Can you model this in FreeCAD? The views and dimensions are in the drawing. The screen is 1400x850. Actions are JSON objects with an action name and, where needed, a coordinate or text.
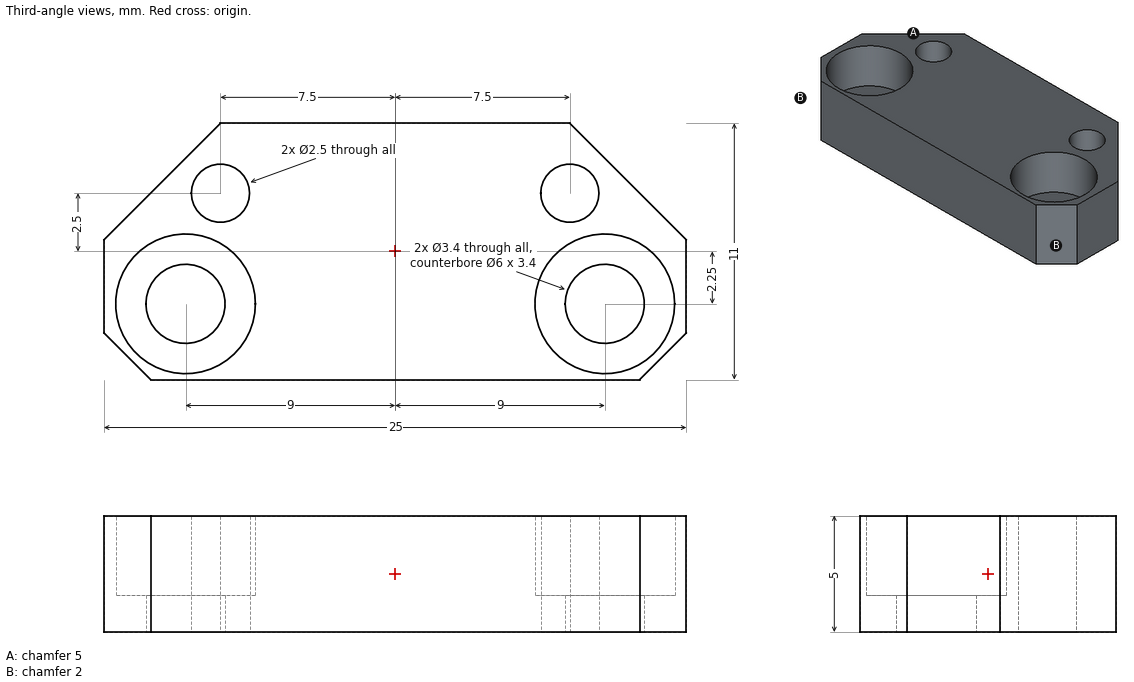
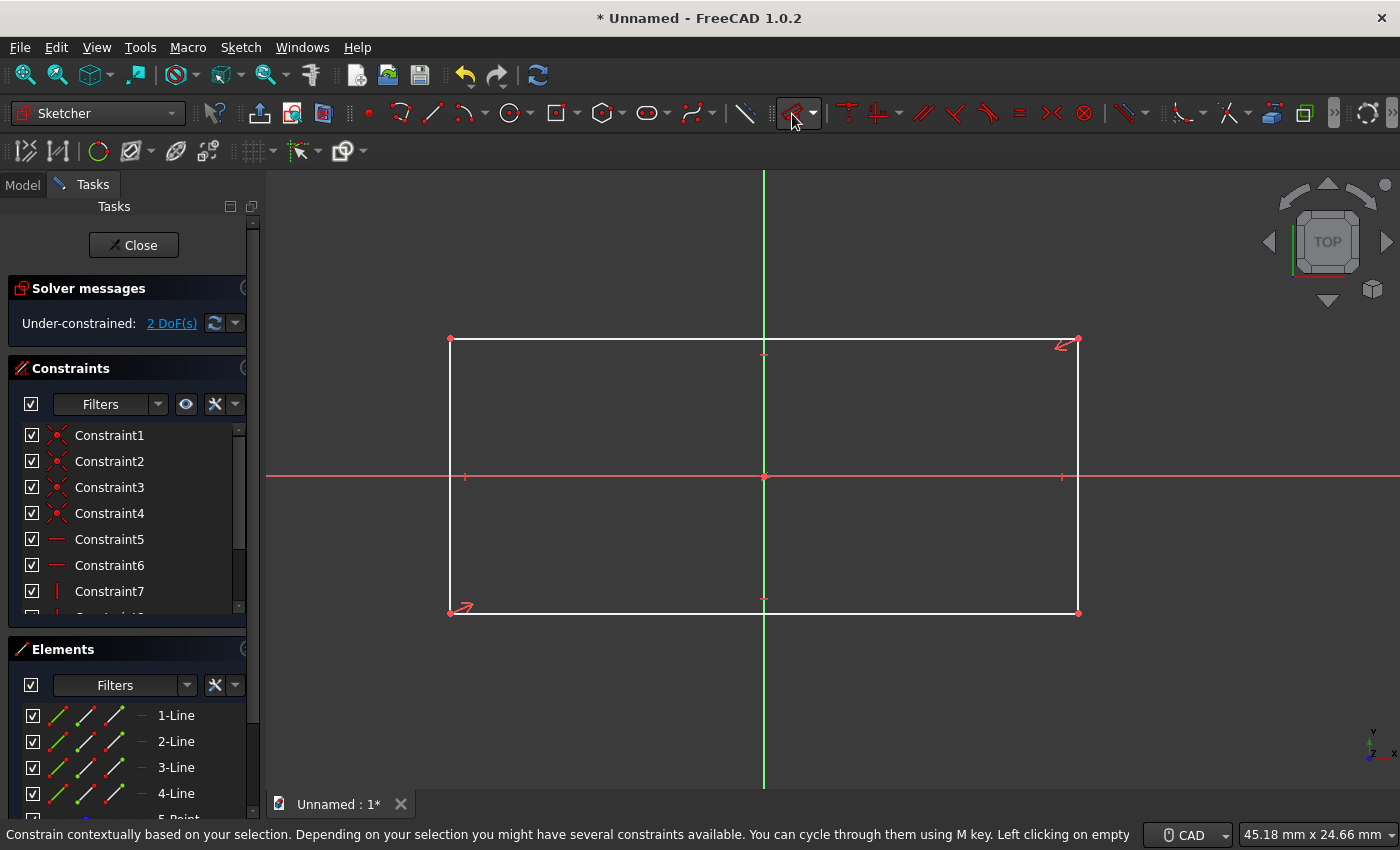
{"action": "left_click", "coordinate": [639, 614]}
{"action": "left_click", "coordinate": [620, 648]}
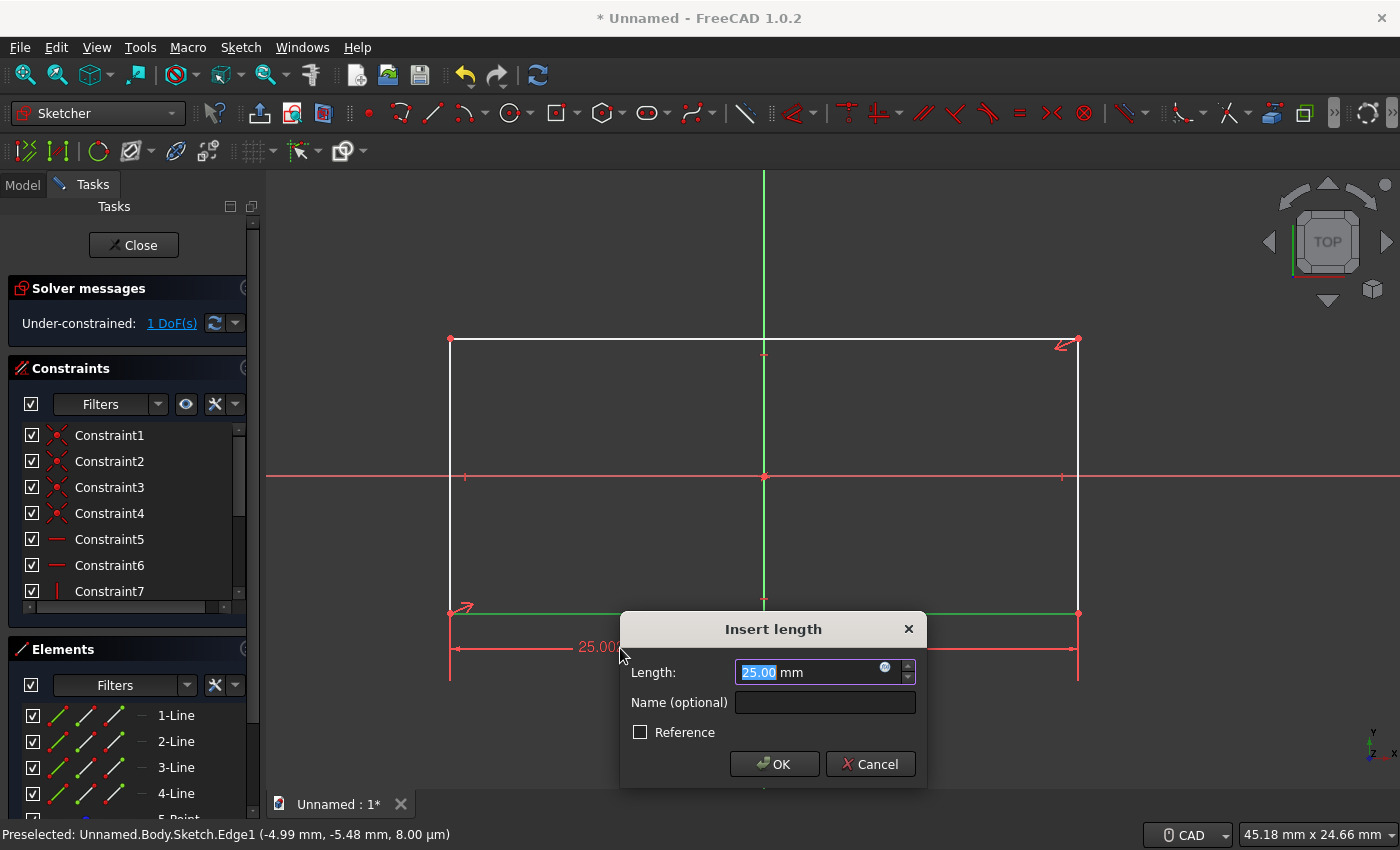
{"action": "type", "text": "25"}
{"action": "key", "text": "Return"}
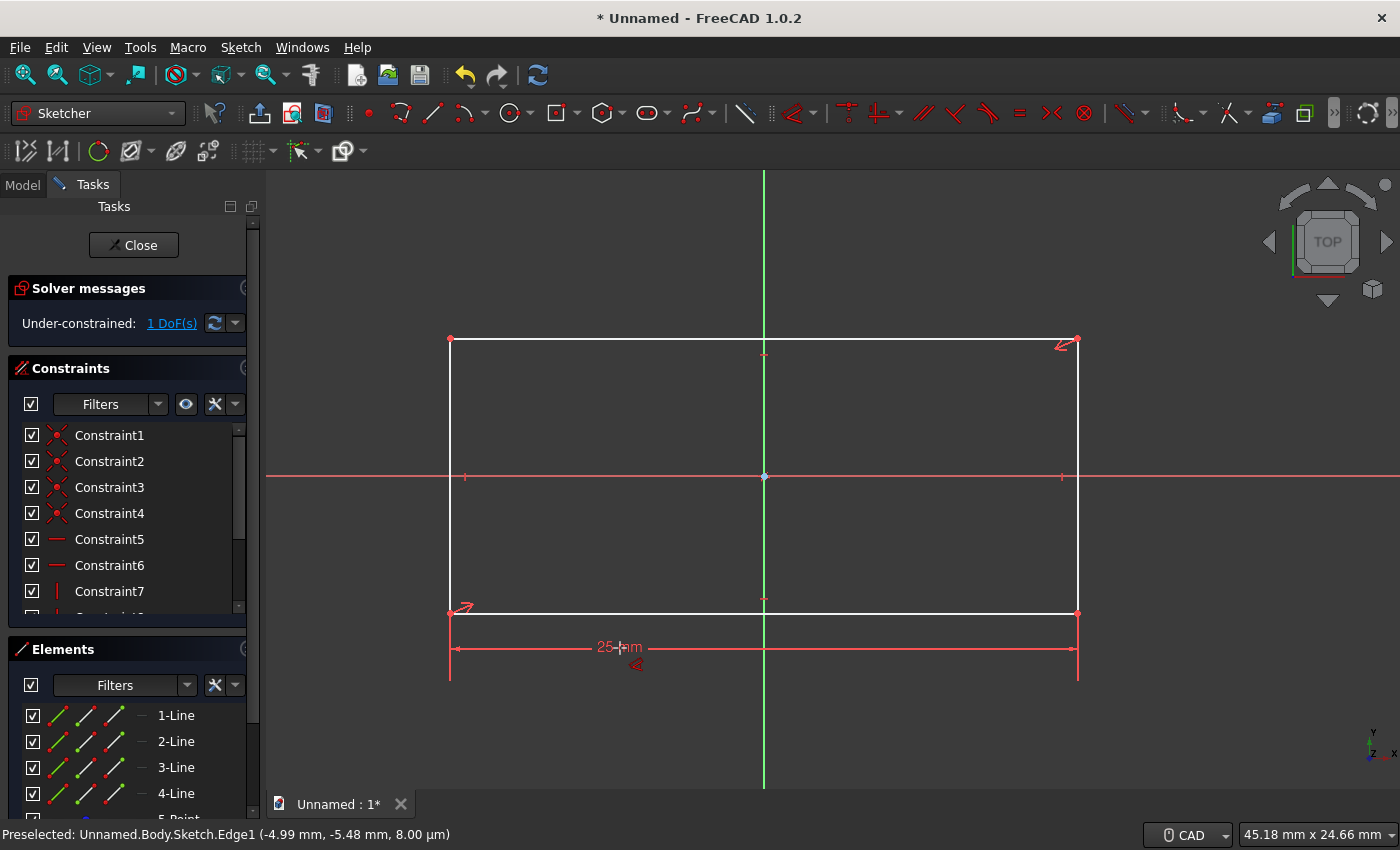
{"action": "left_click", "coordinate": [1078, 531]}
{"action": "left_click", "coordinate": [1112, 413]}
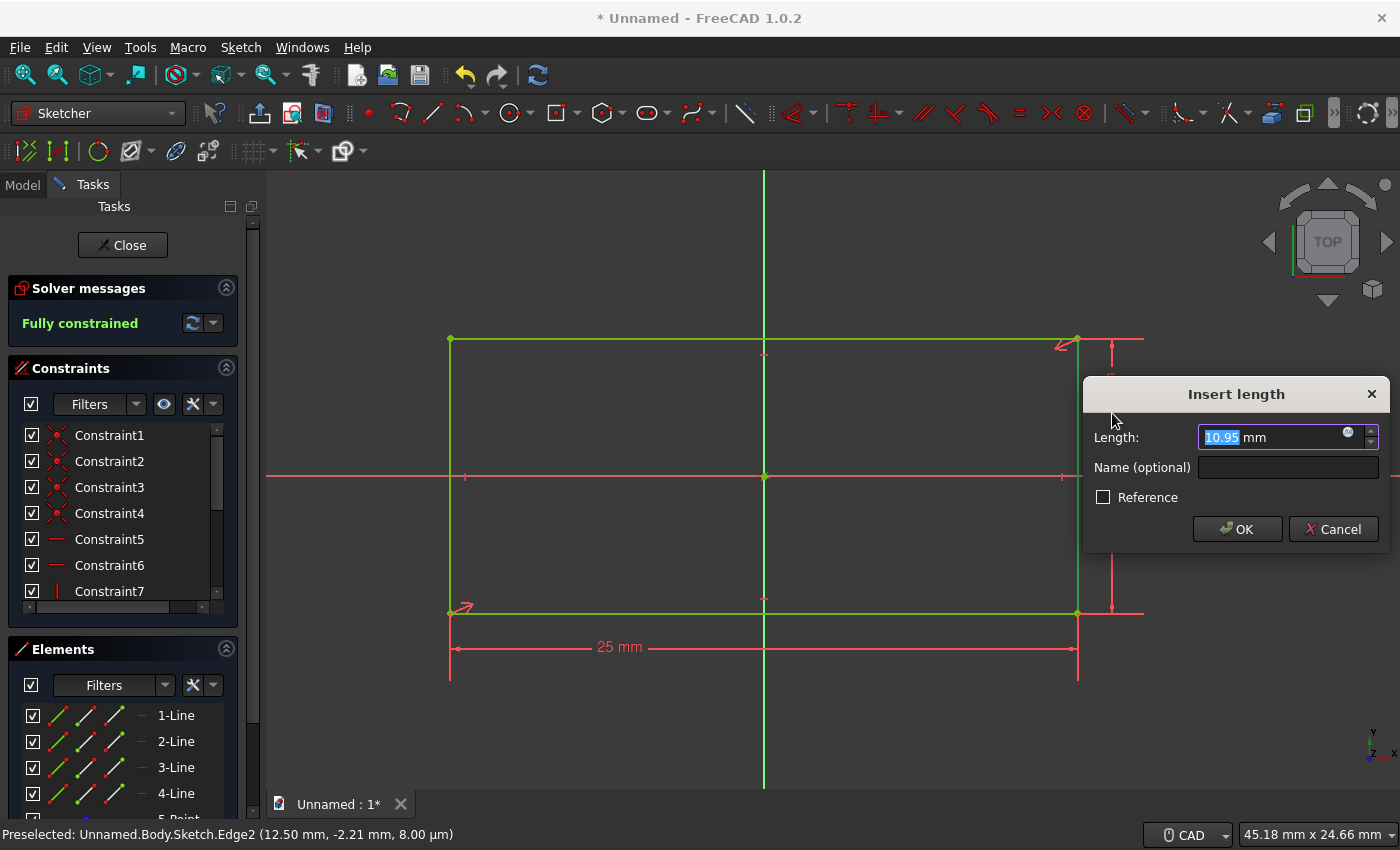
{"action": "type", "text": "11"}
{"action": "key", "text": "Return"}
{"action": "key", "text": "Escape"}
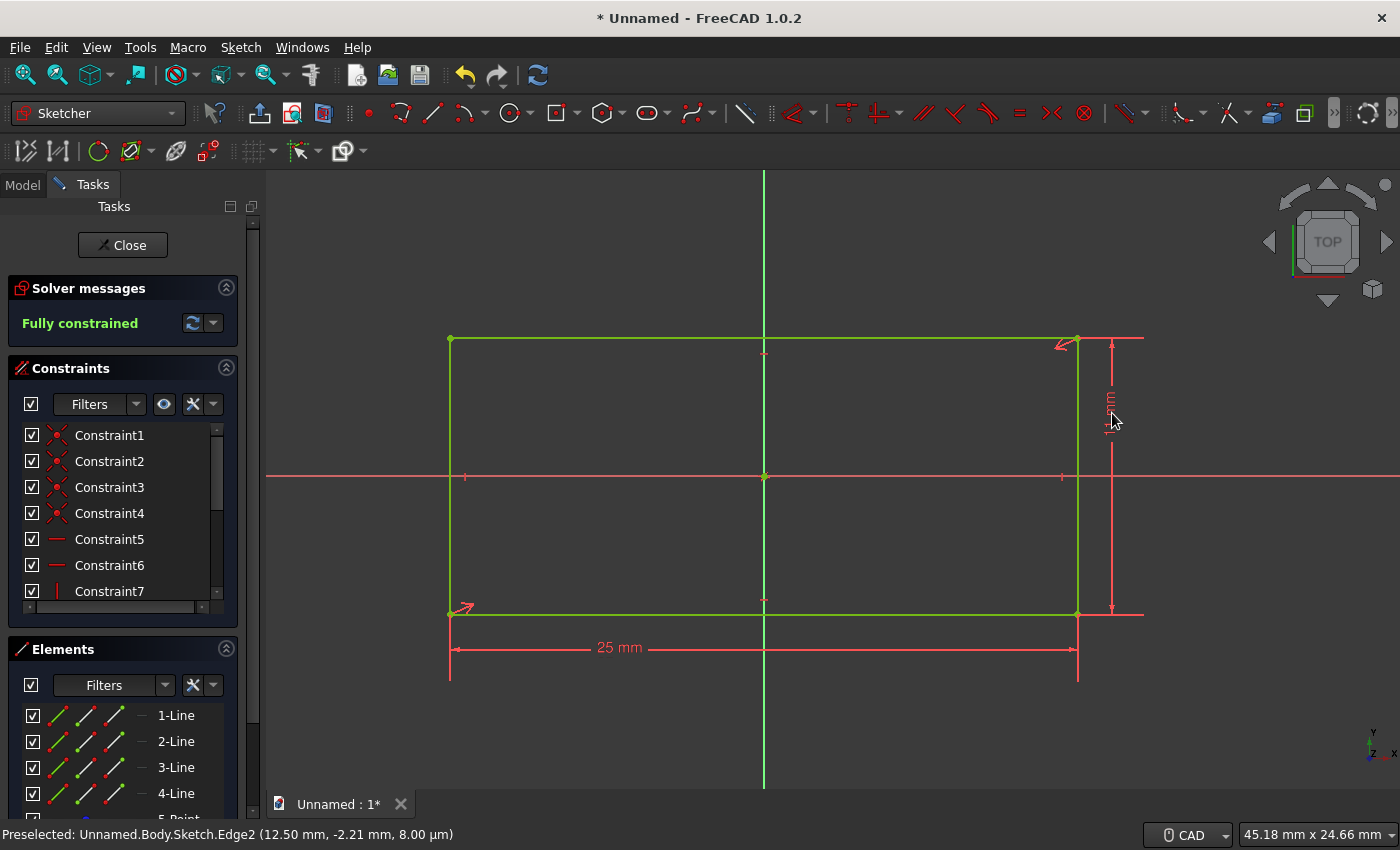
{"action": "left_click", "coordinate": [123, 245]}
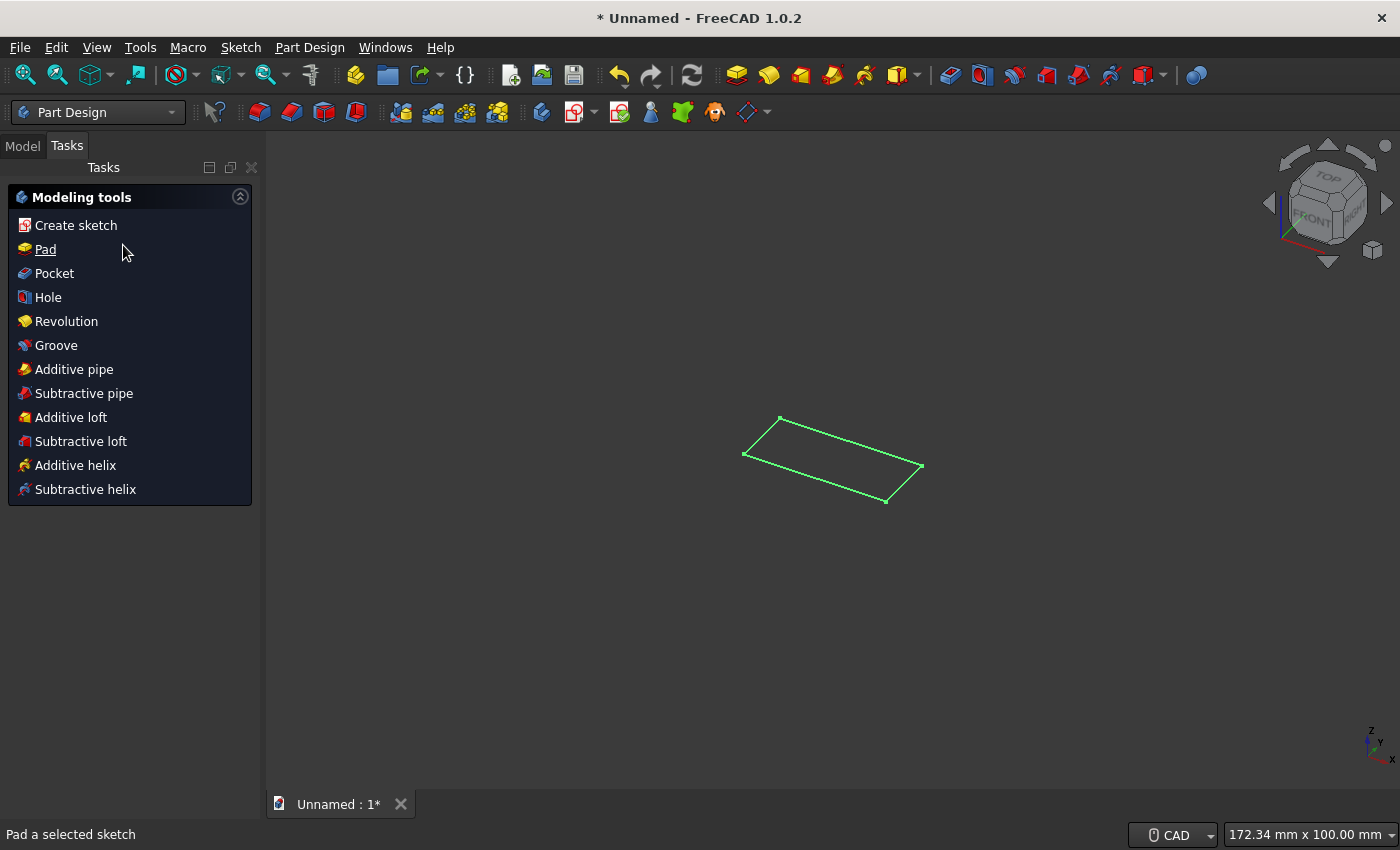
{"action": "left_click", "coordinate": [738, 76]}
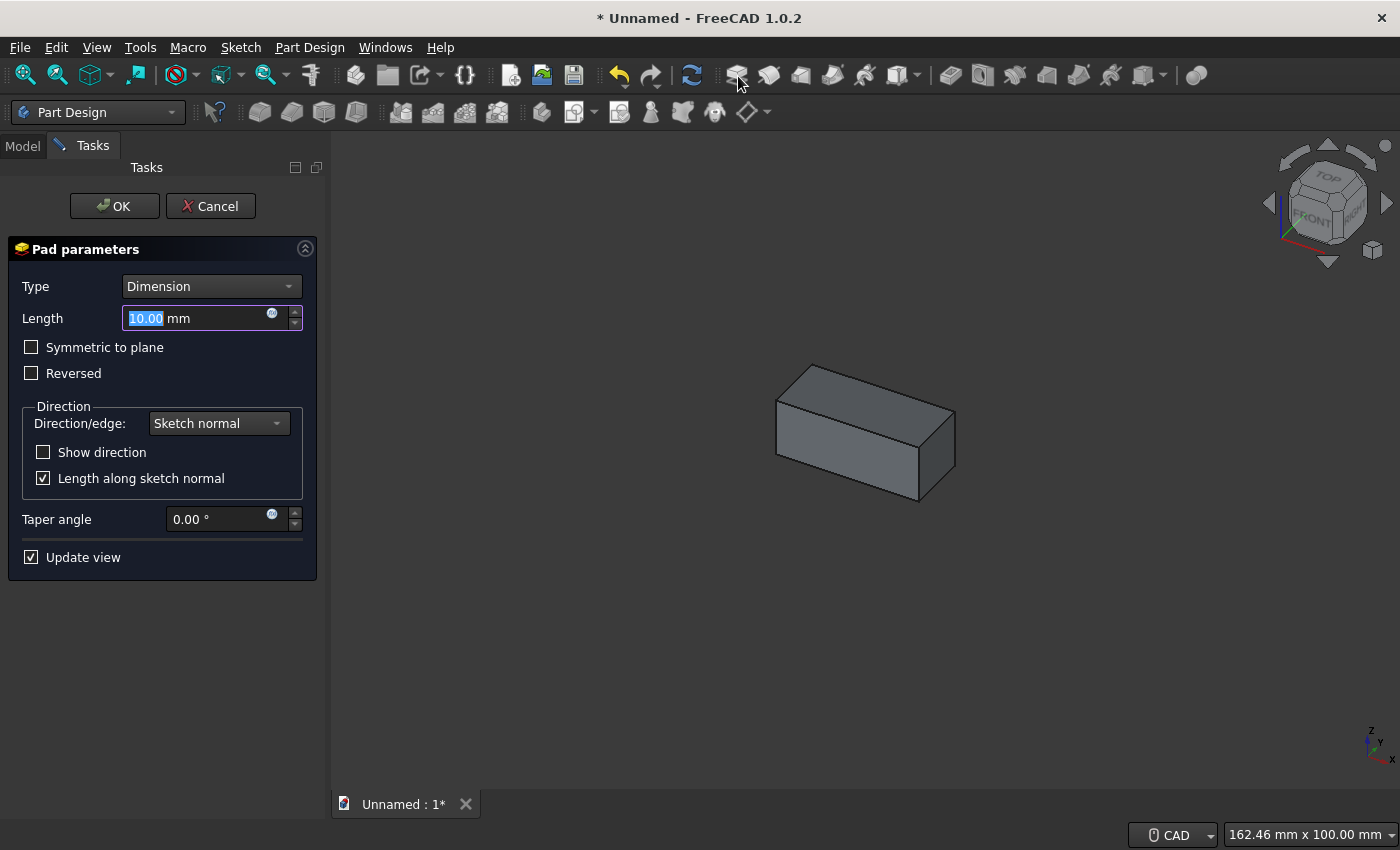
{"action": "type", "text": "5"}
{"action": "key", "text": "Tab"}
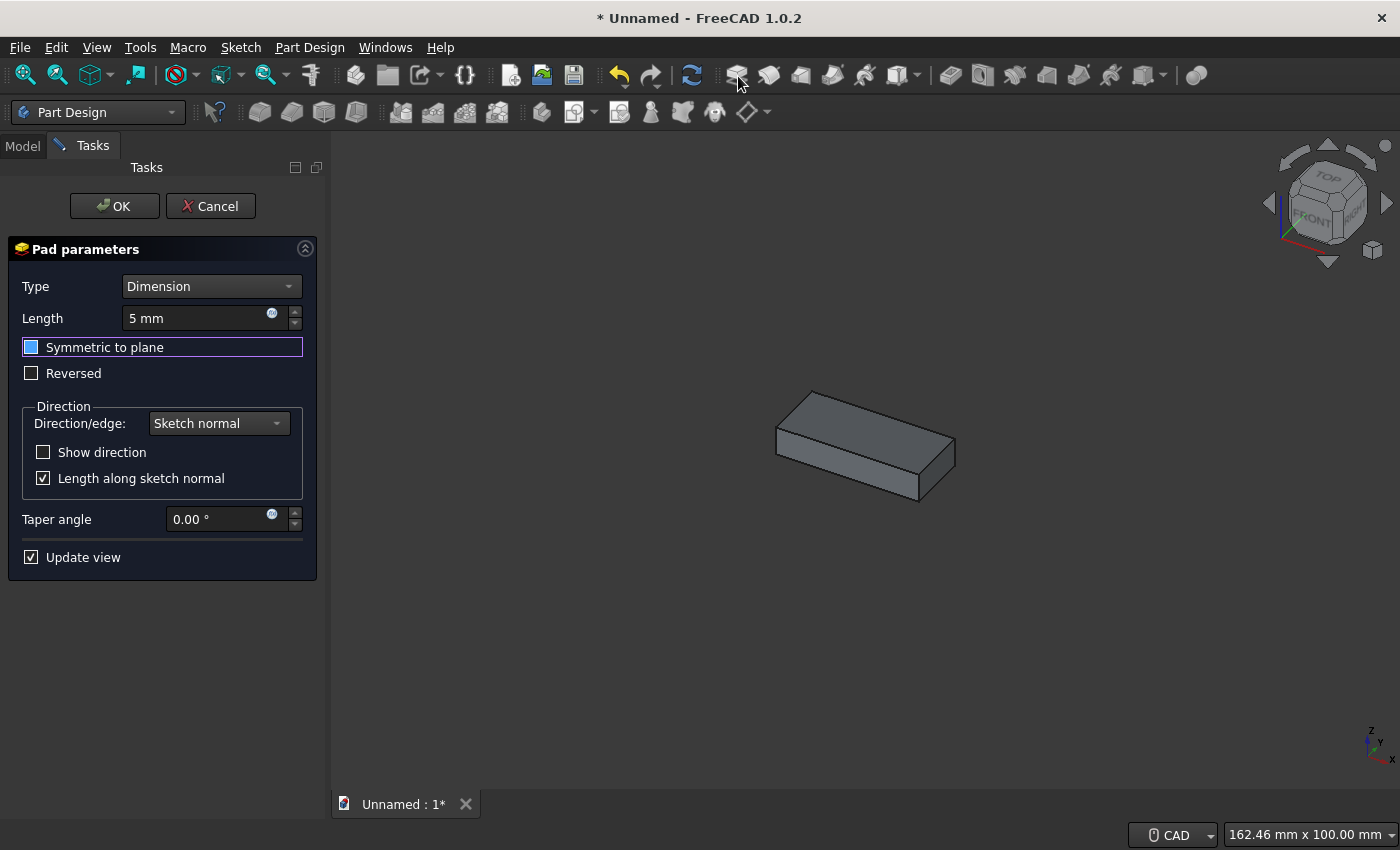
{"action": "left_click", "coordinate": [30, 347]}